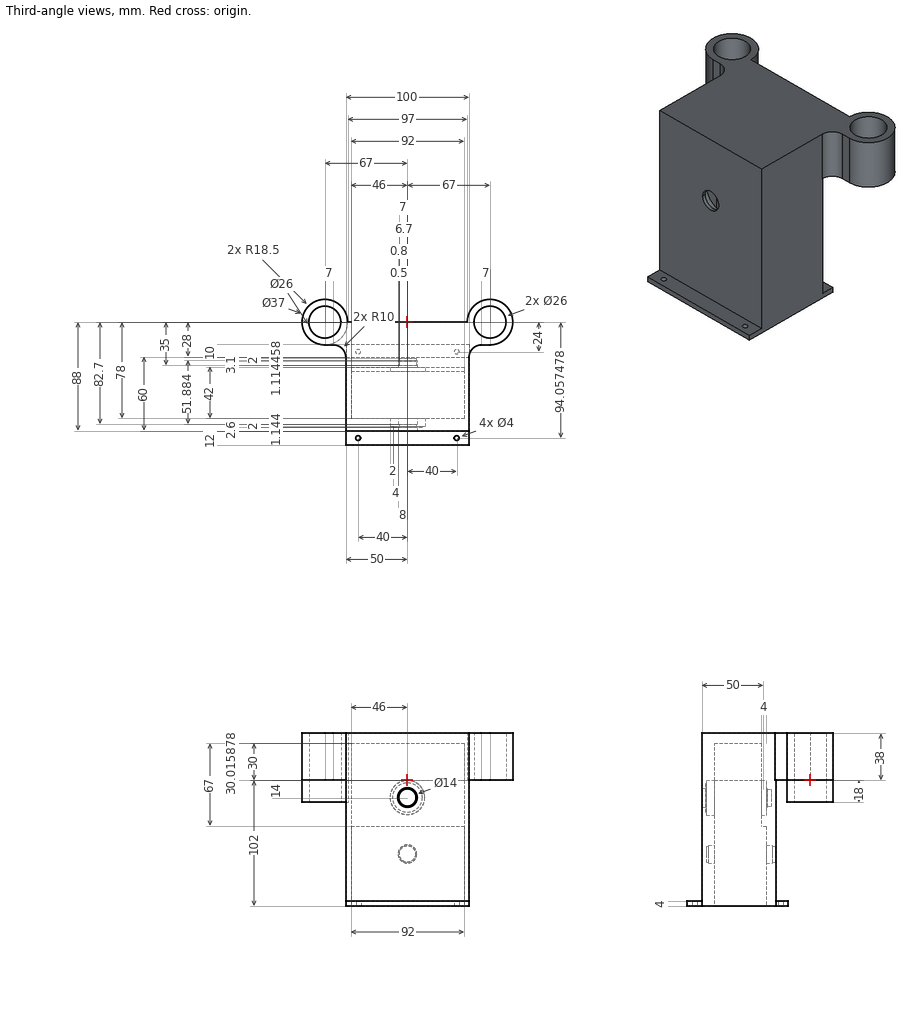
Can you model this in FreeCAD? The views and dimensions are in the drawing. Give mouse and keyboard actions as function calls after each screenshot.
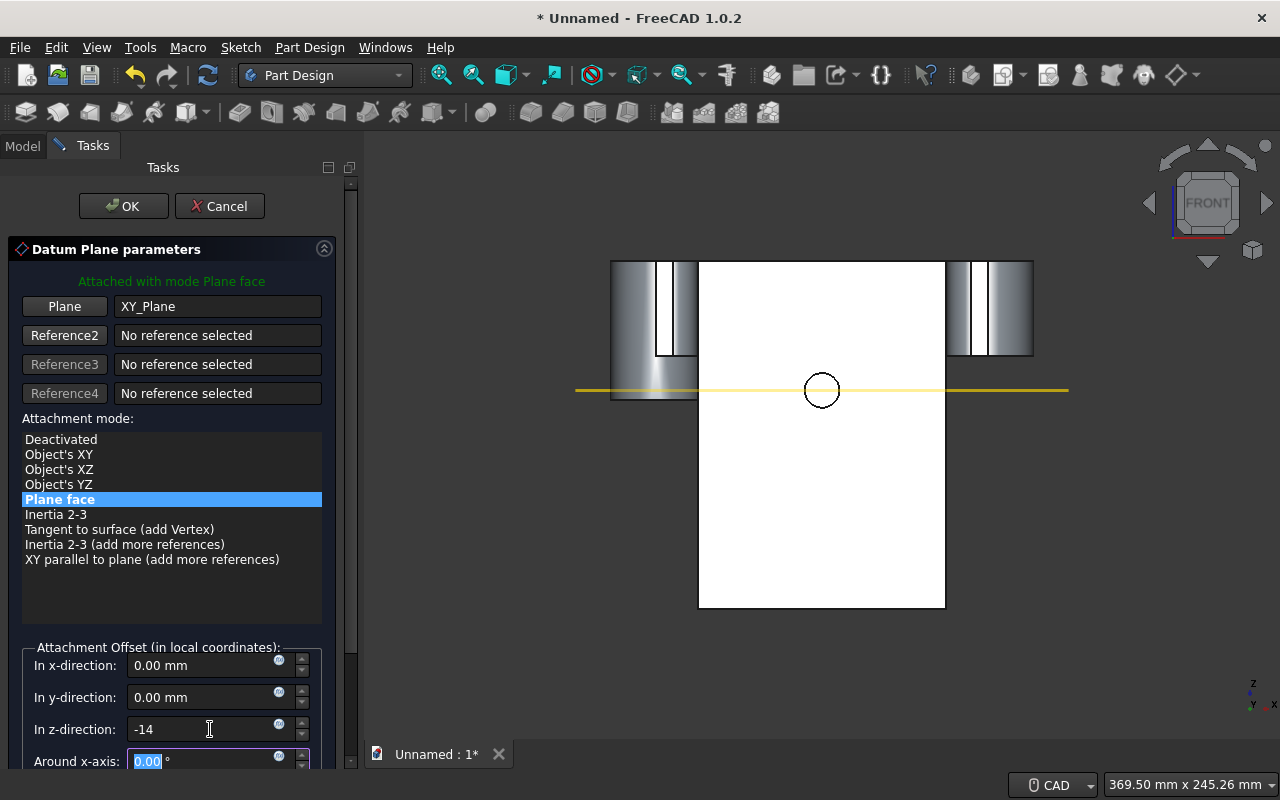
click(124, 206)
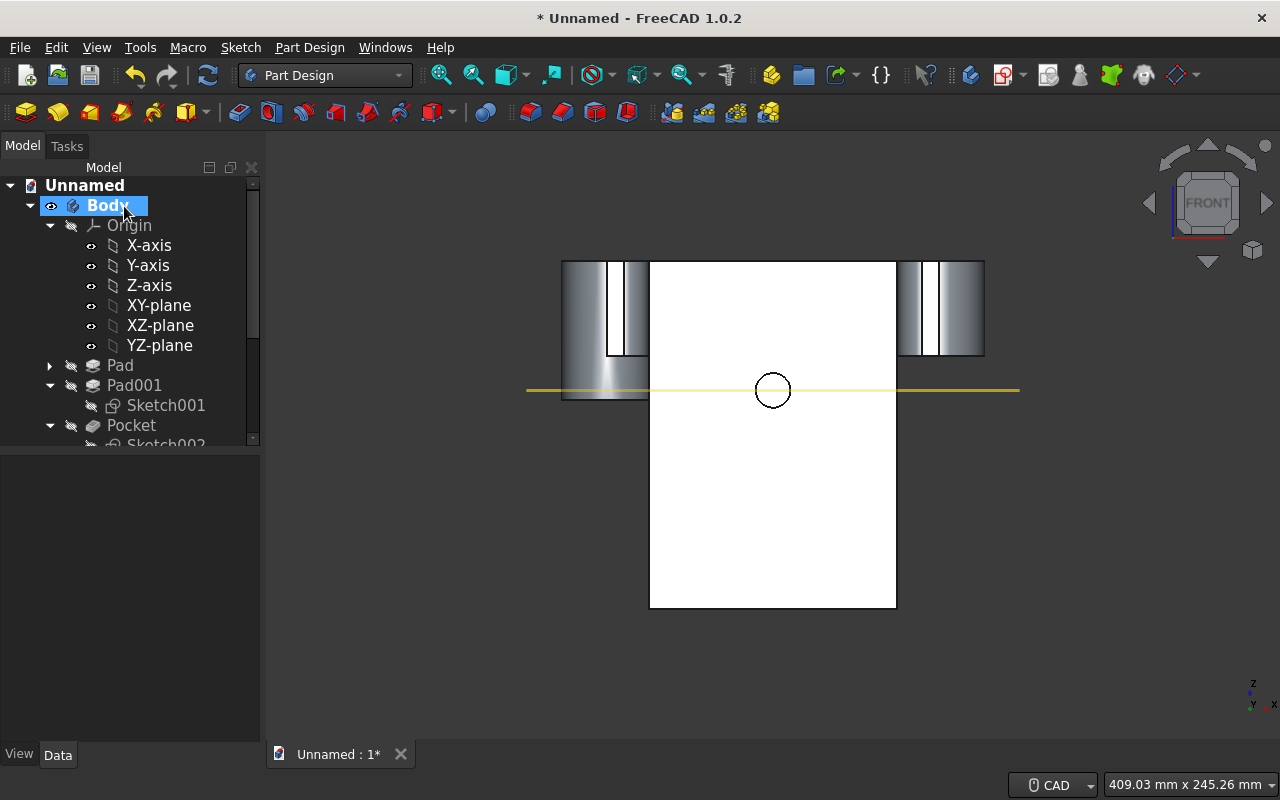
scroll(100, 321, down, 3)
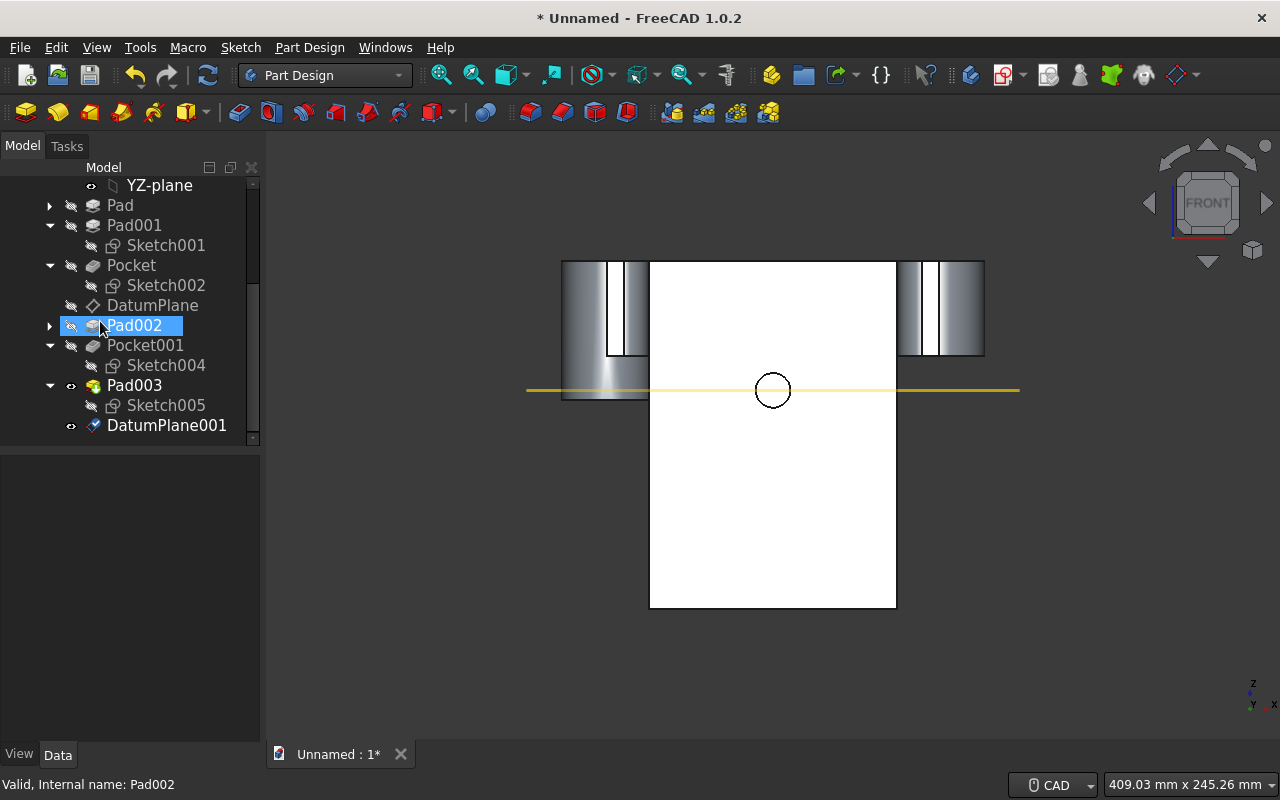
click(116, 426)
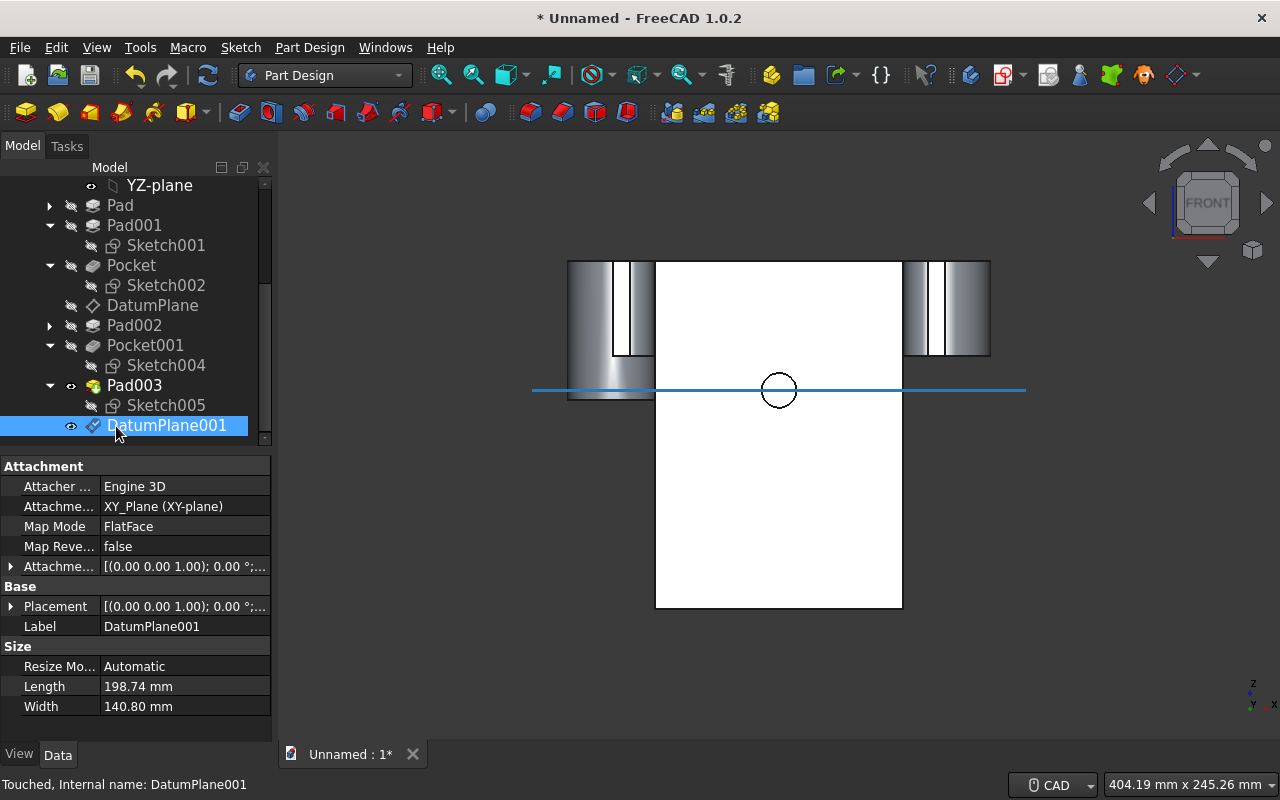
click(1004, 76)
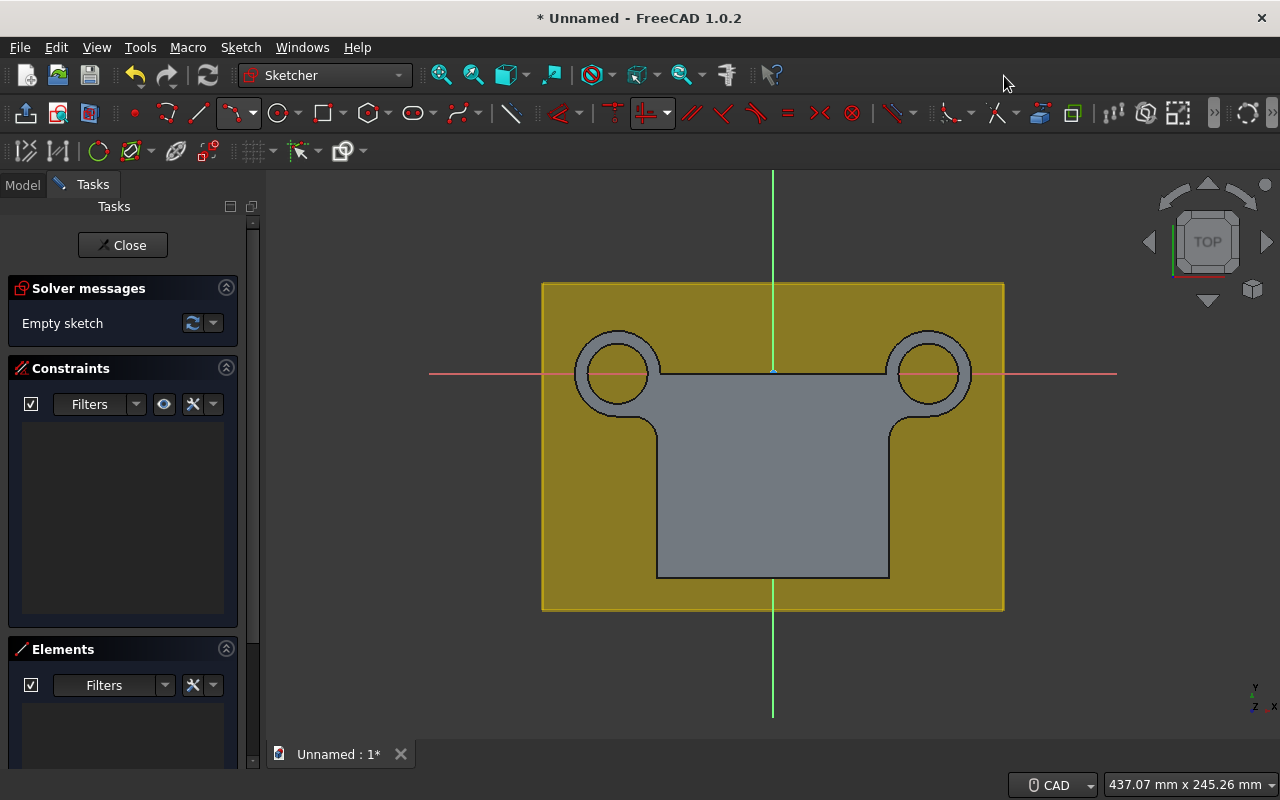
key(q)
key(s)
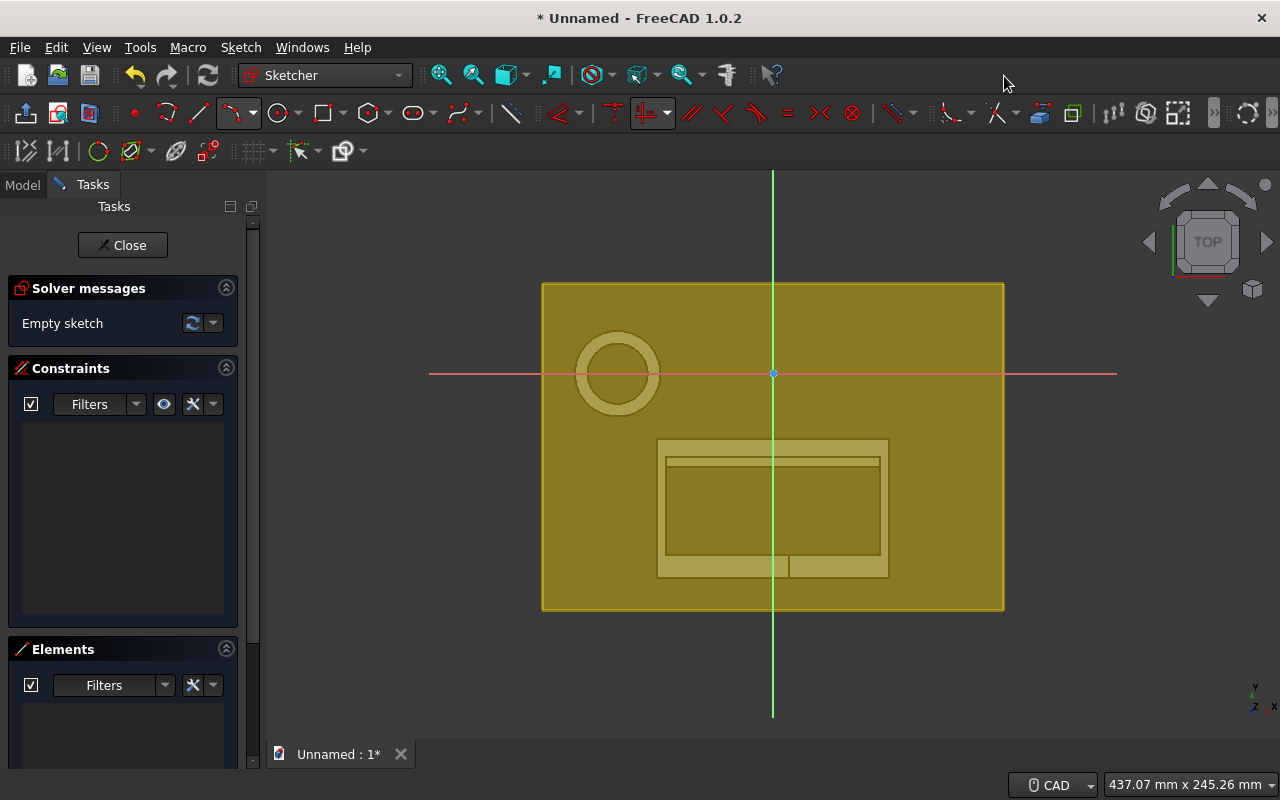
scroll(820, 502, up, 3)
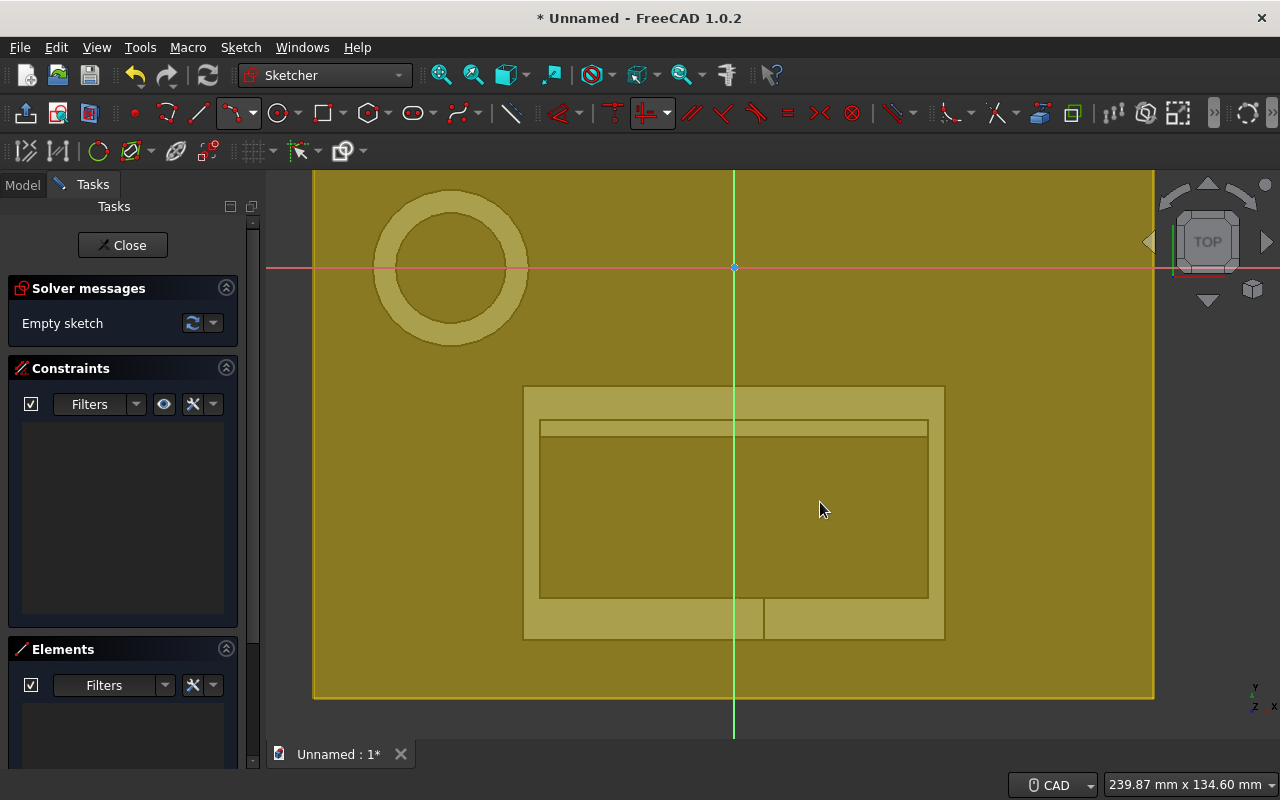
click(168, 114)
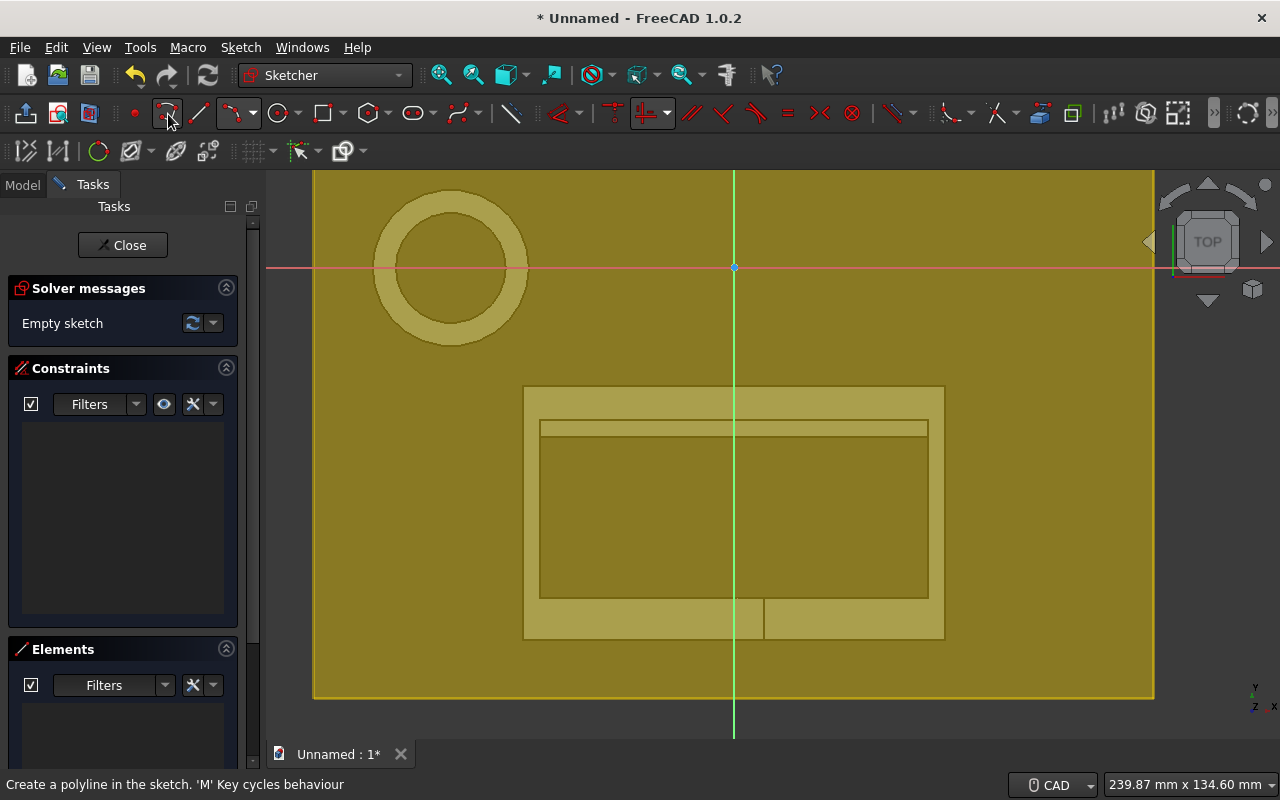
click(734, 403)
click(704, 403)
click(704, 416)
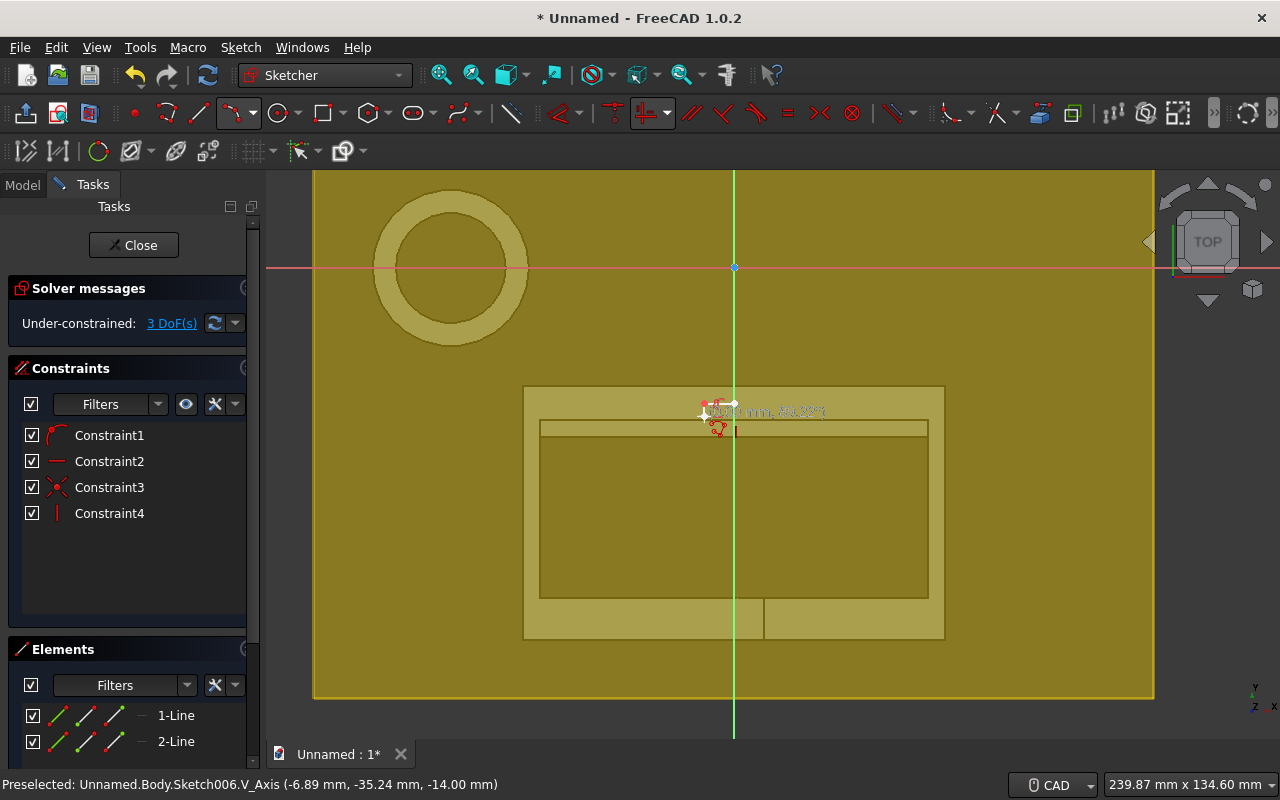
scroll(702, 416, up, 11)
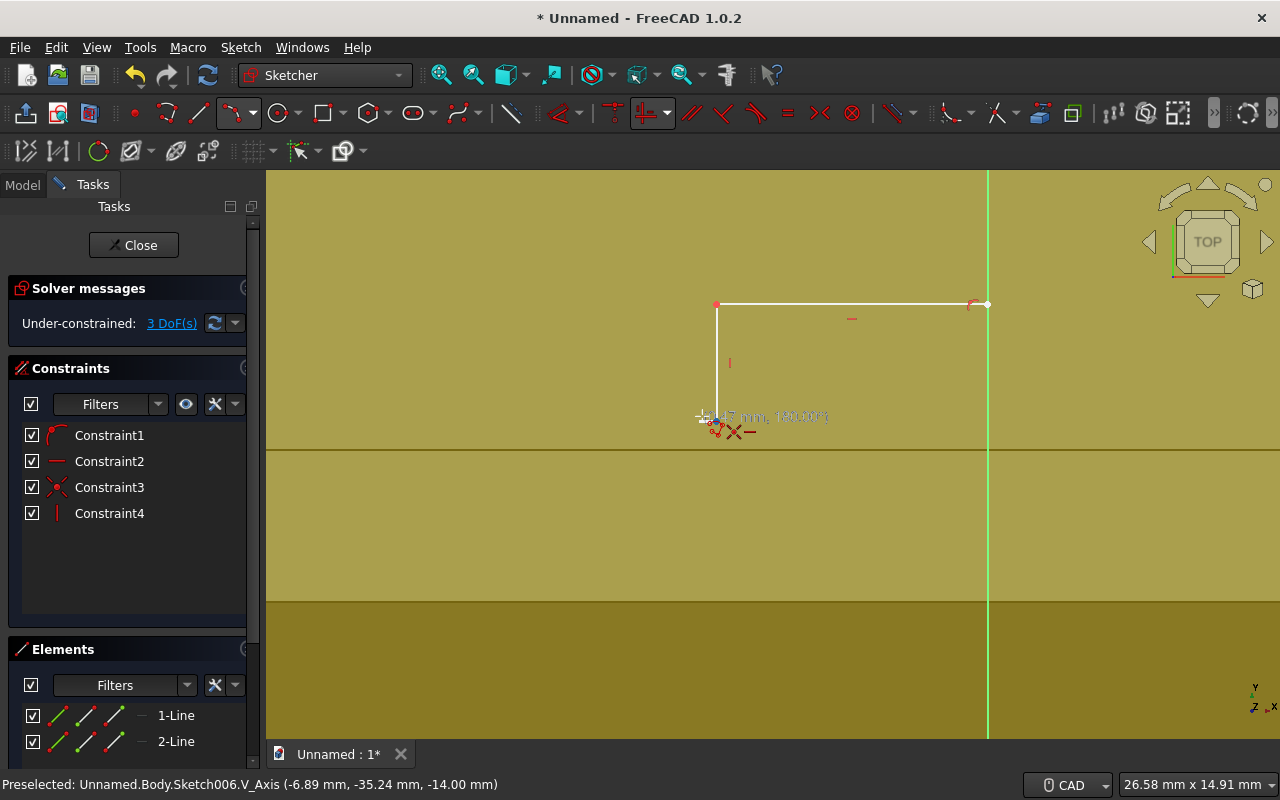
click(701, 413)
click(701, 454)